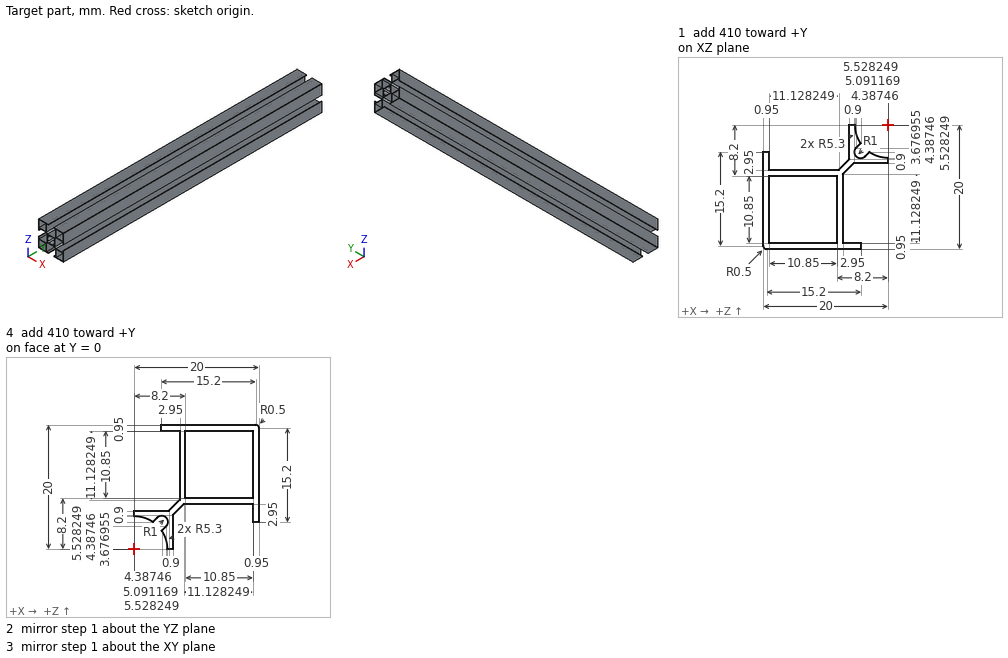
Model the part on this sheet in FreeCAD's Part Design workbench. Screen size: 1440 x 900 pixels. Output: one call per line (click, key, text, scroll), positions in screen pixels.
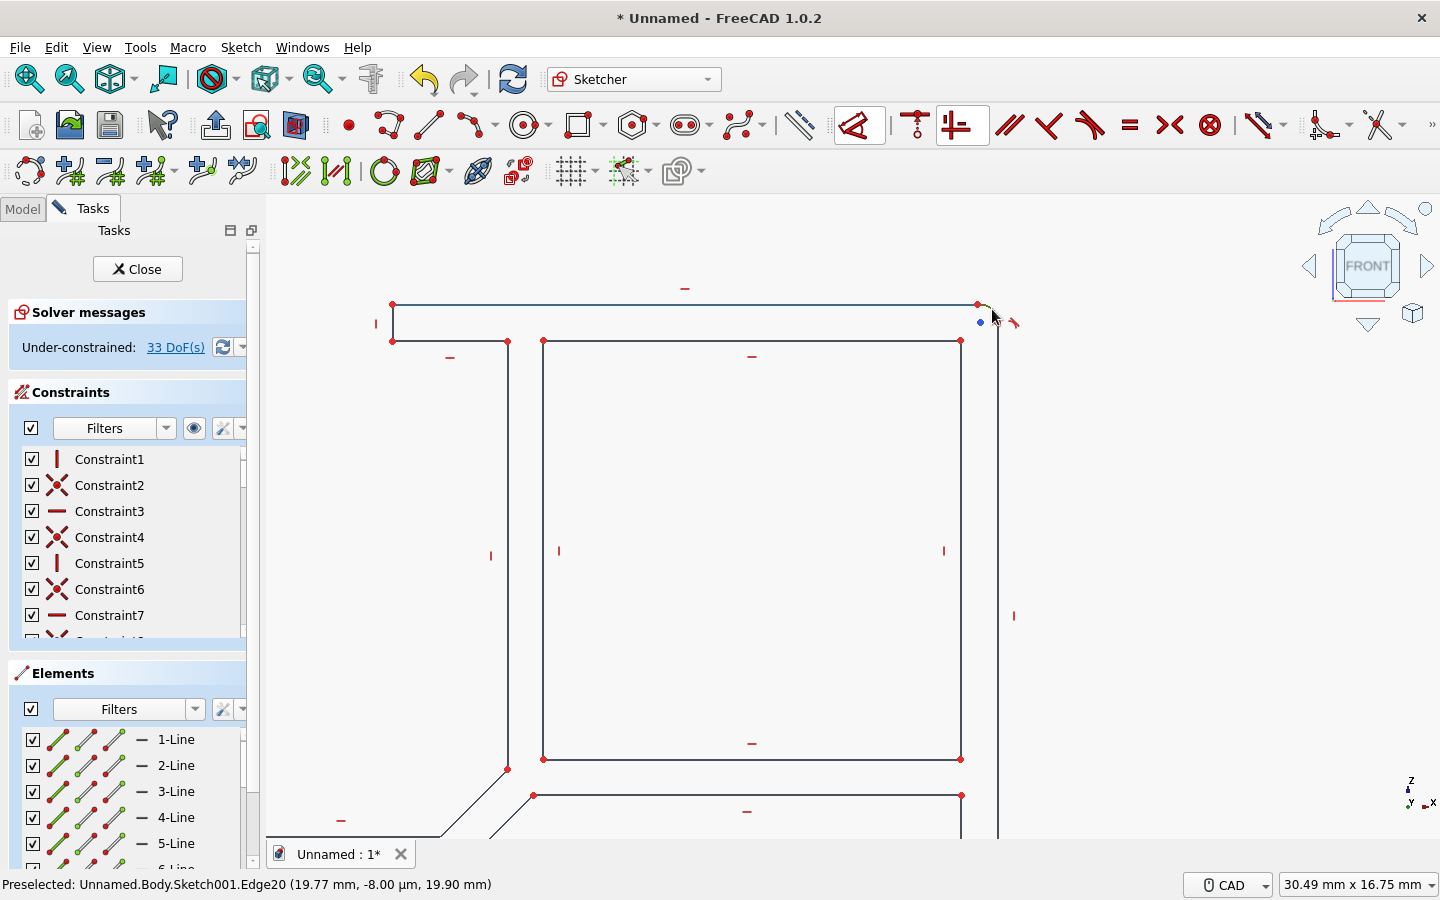
click(1090, 126)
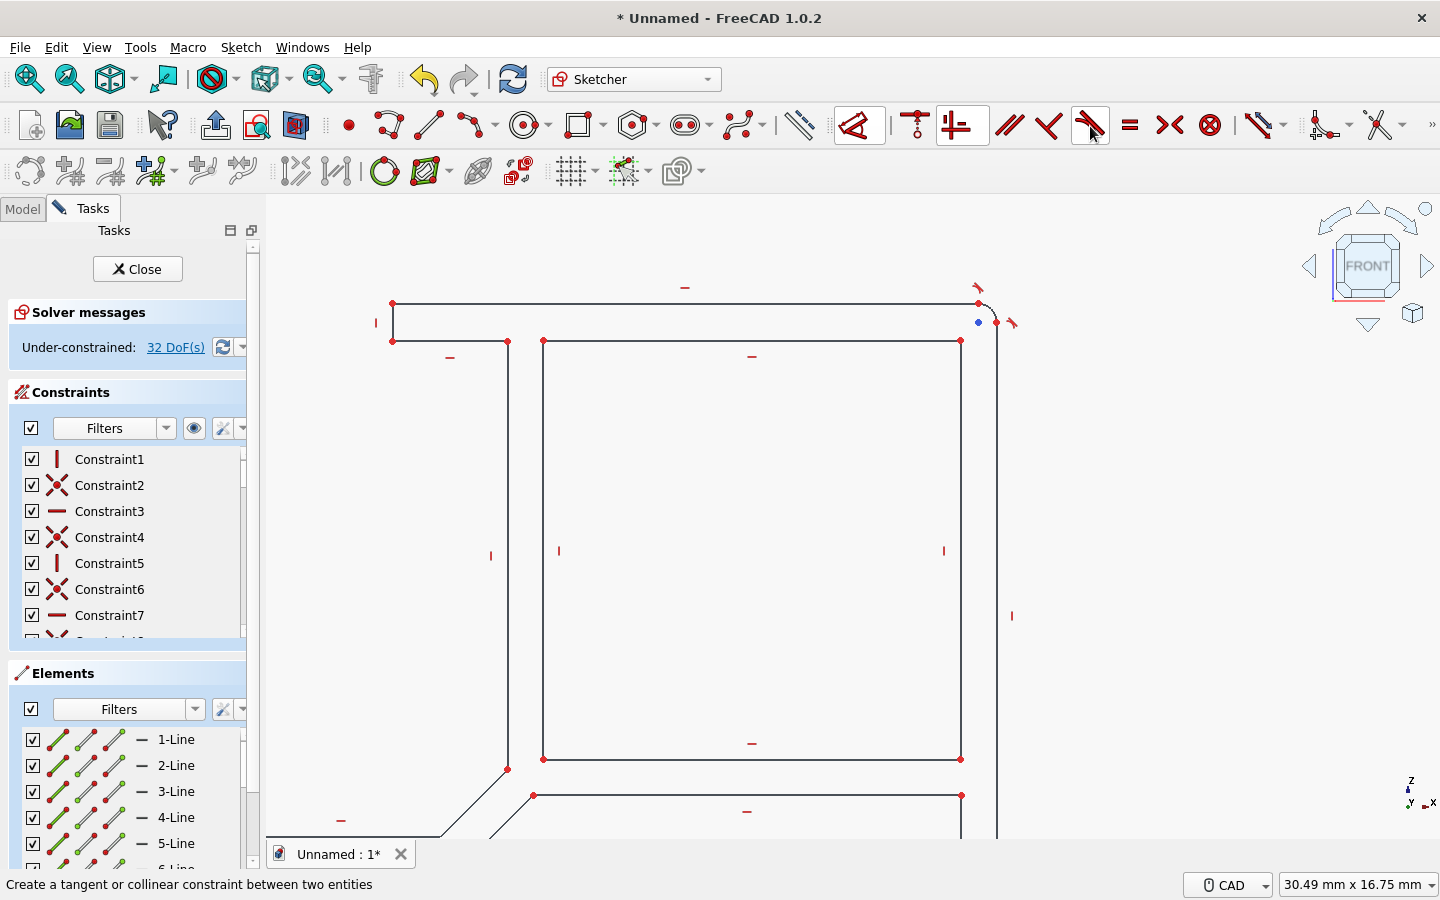
scroll(993, 308, down, 3)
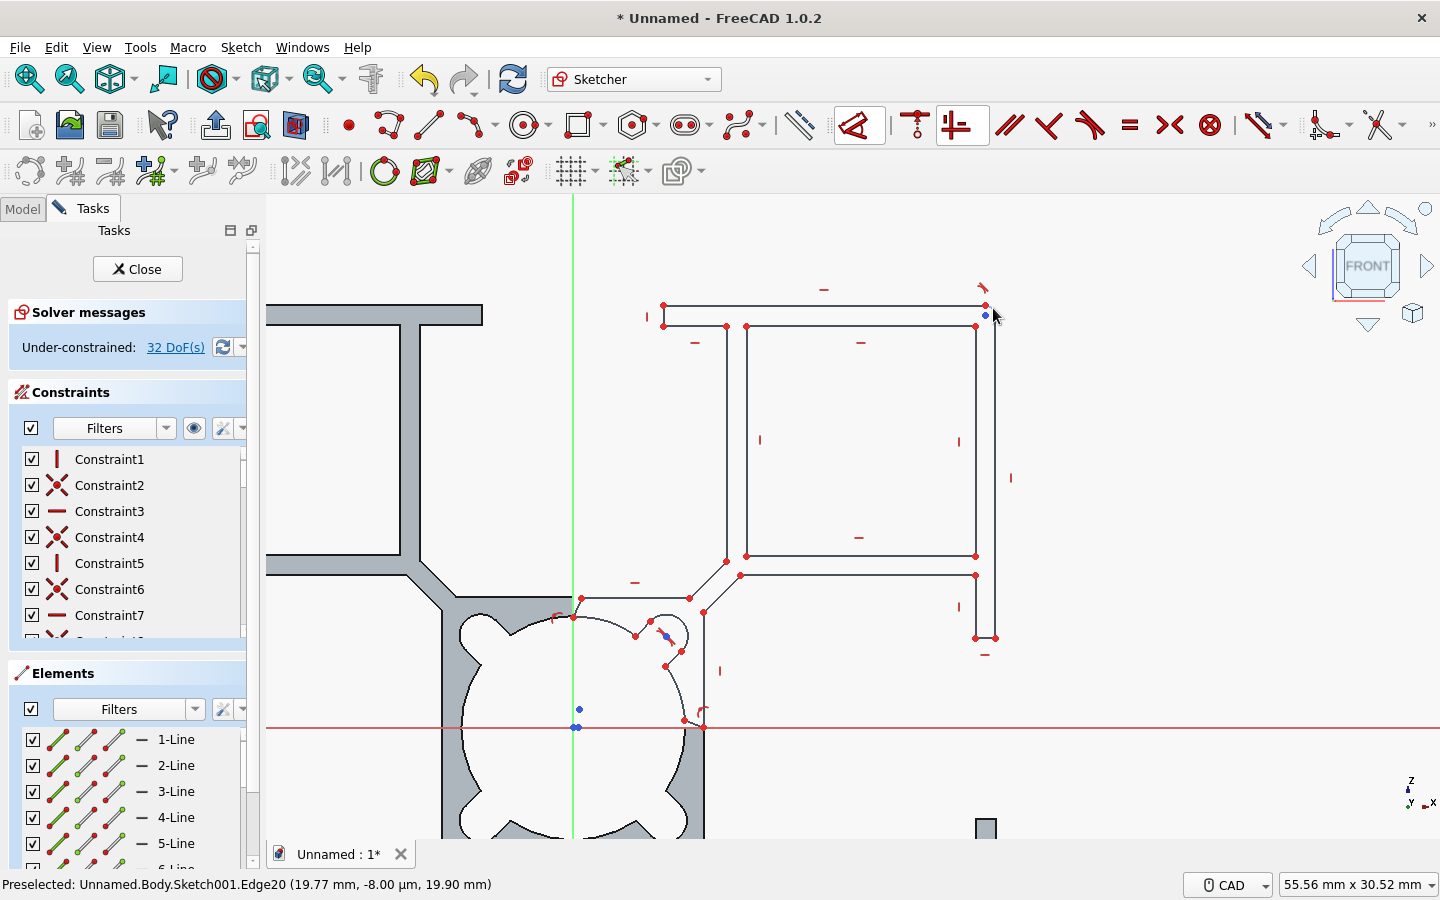
scroll(691, 723, up, 5)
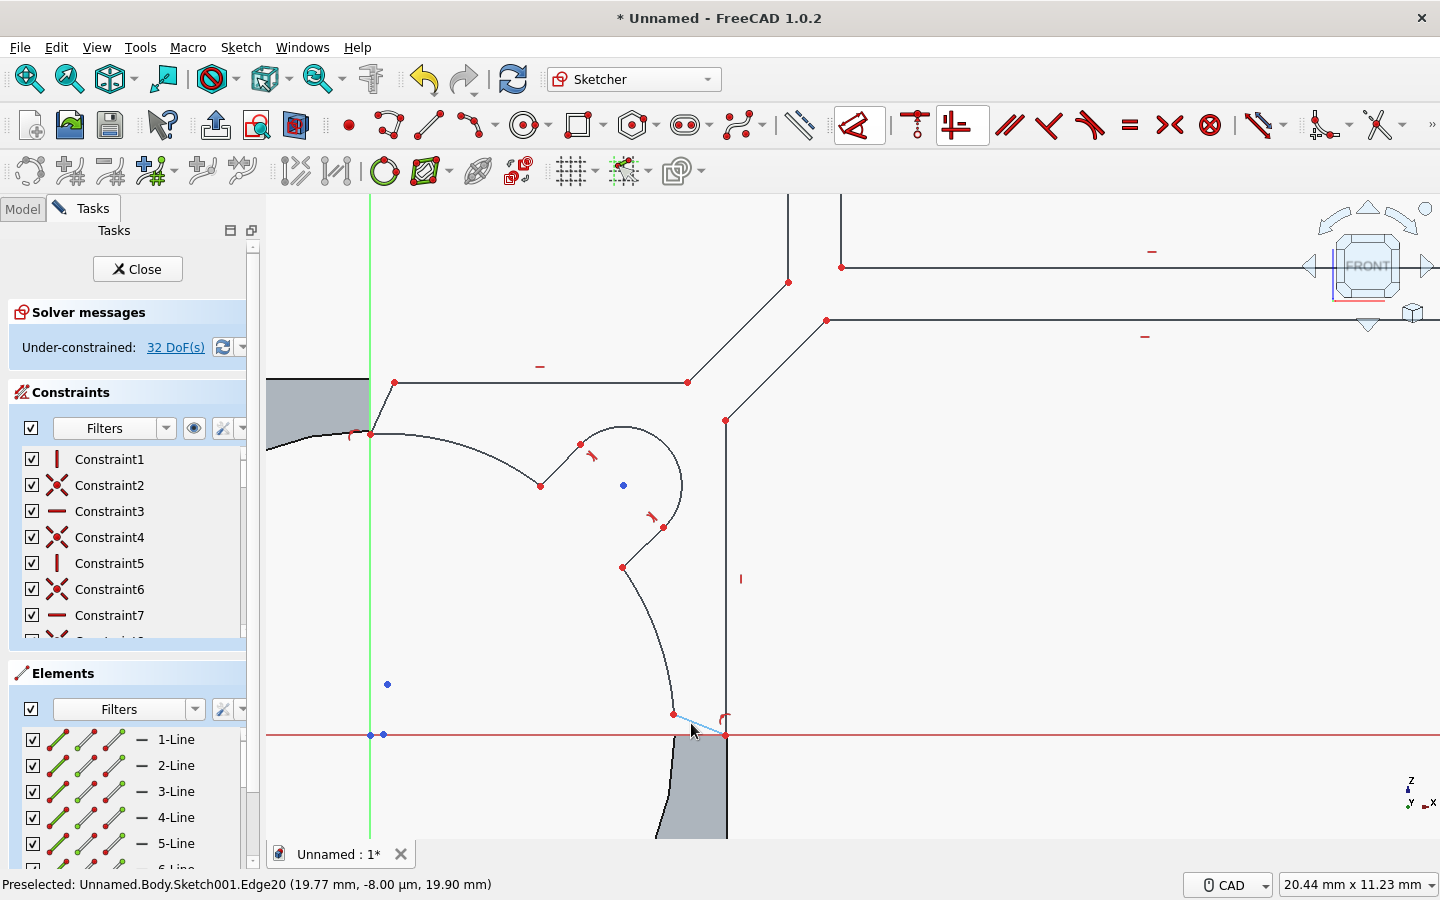
click(689, 721)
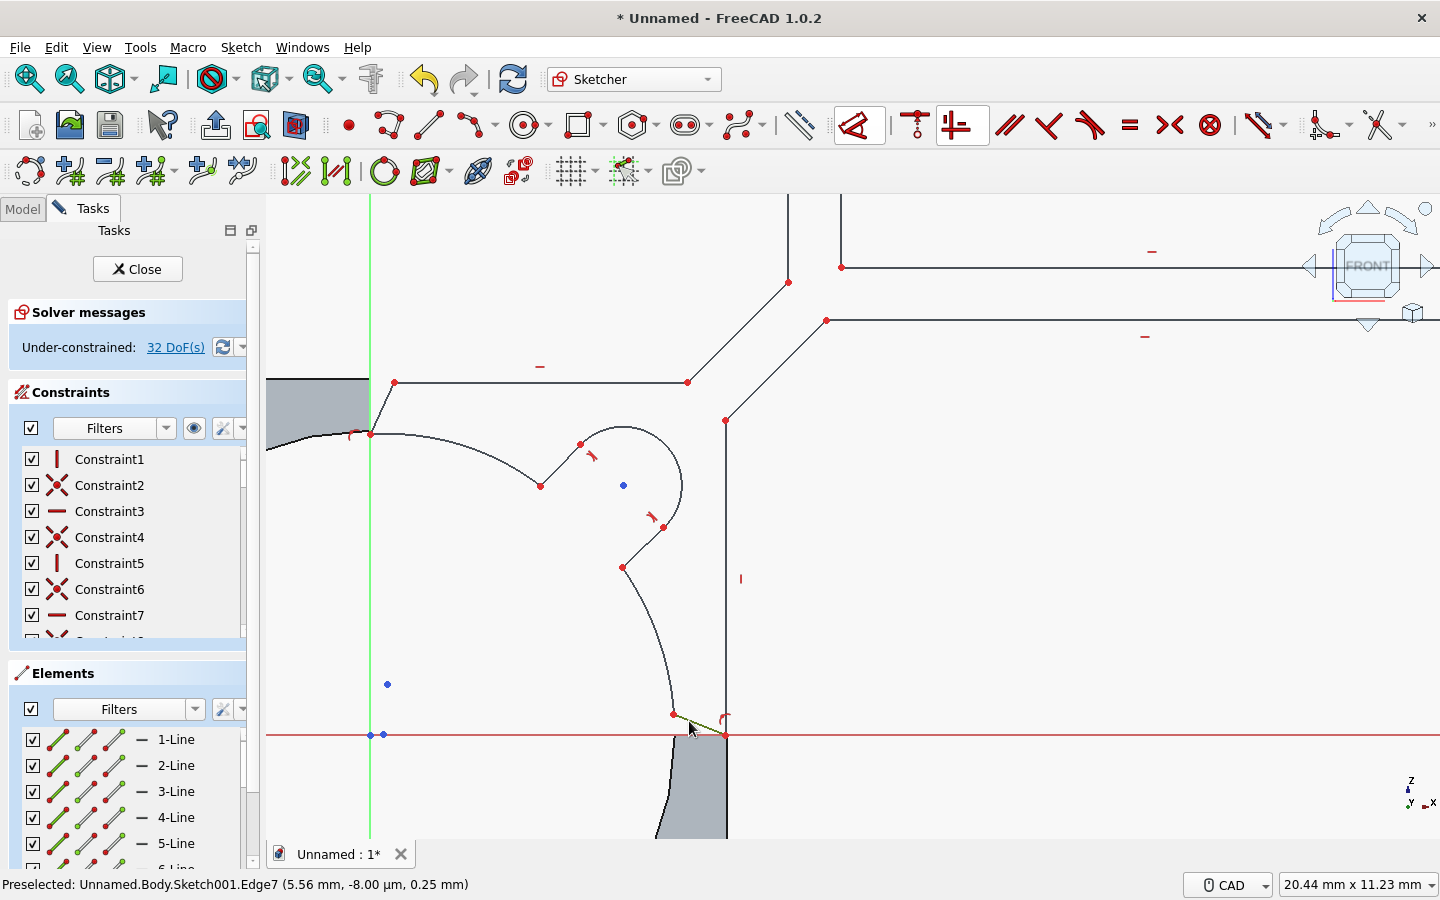
click(984, 126)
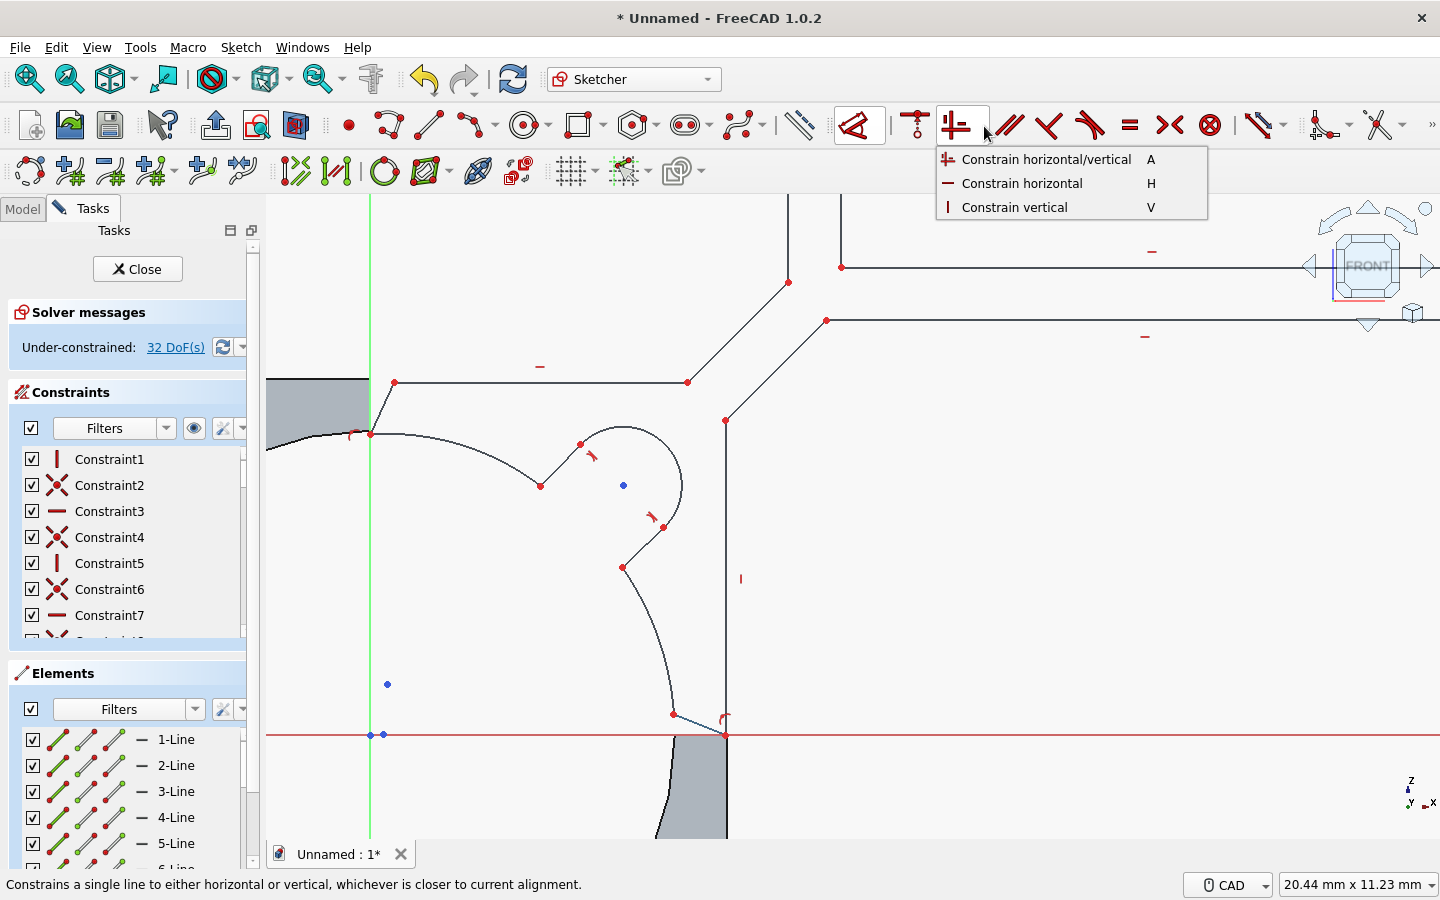
click(1072, 183)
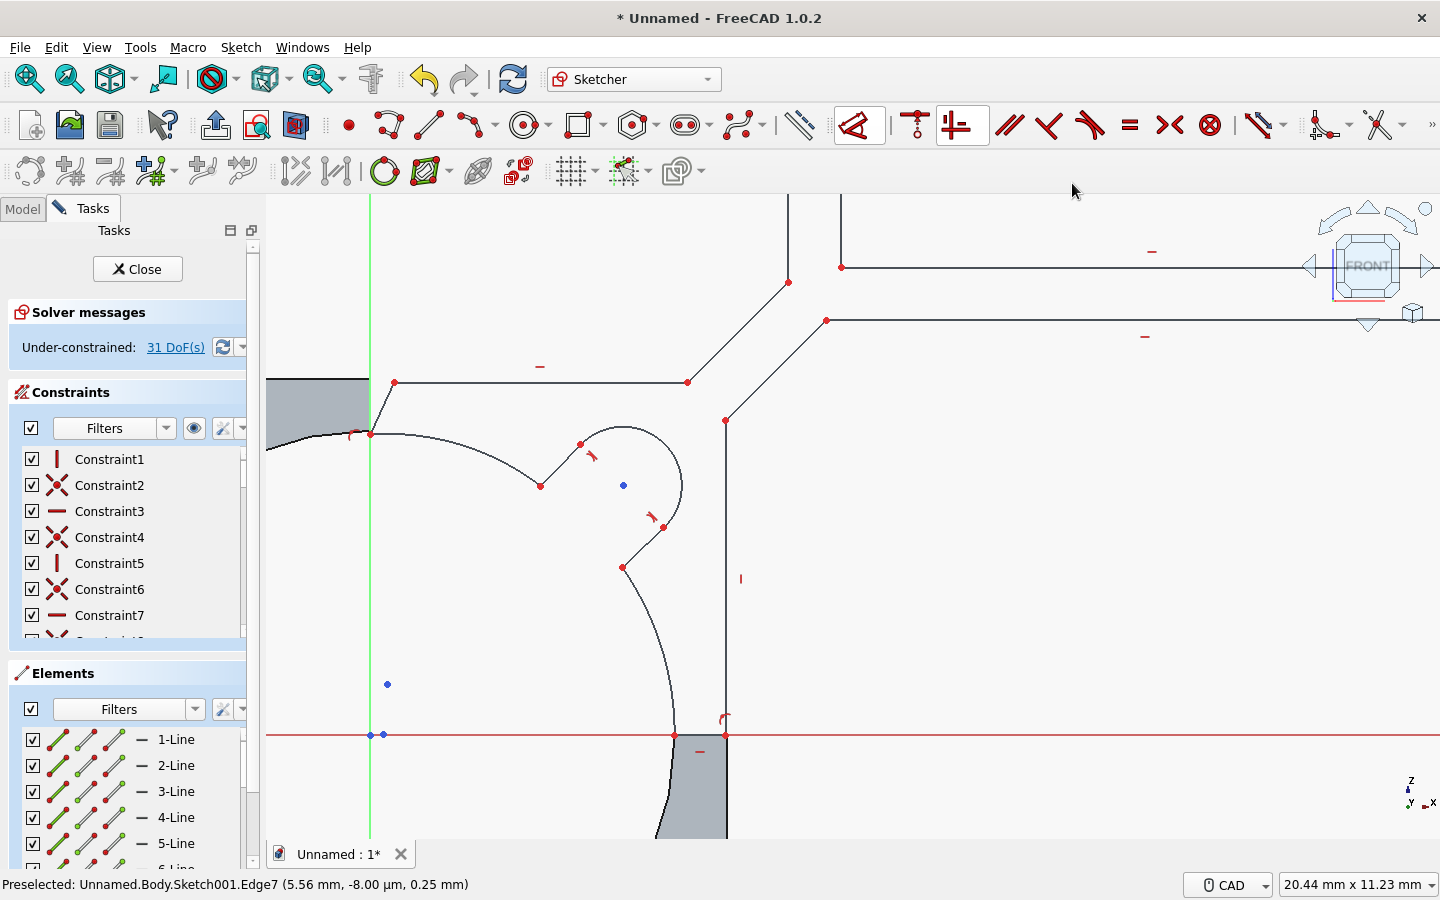
click(387, 398)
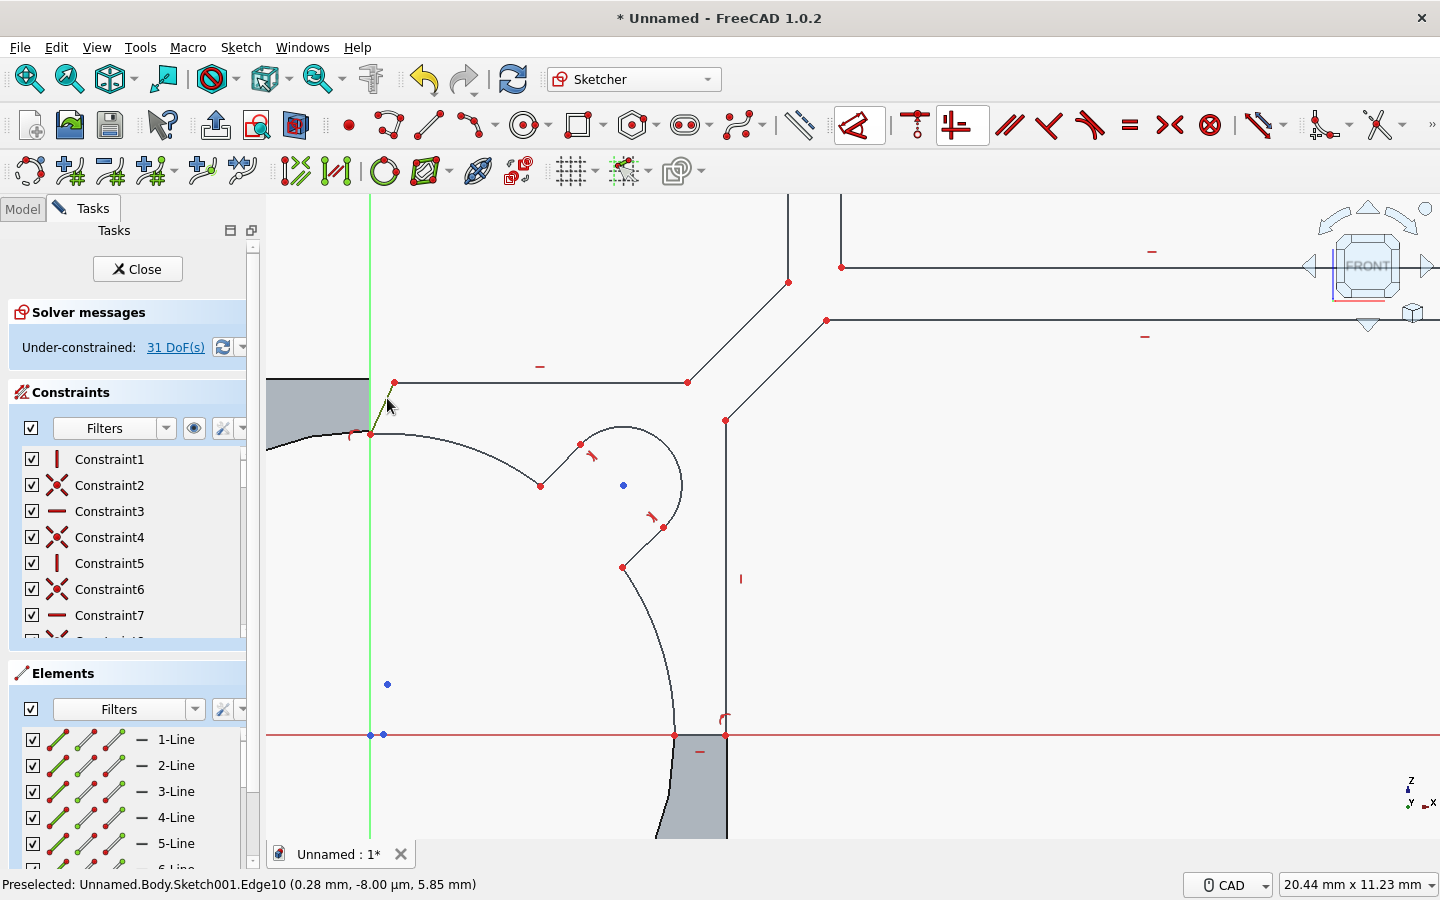
key(v)